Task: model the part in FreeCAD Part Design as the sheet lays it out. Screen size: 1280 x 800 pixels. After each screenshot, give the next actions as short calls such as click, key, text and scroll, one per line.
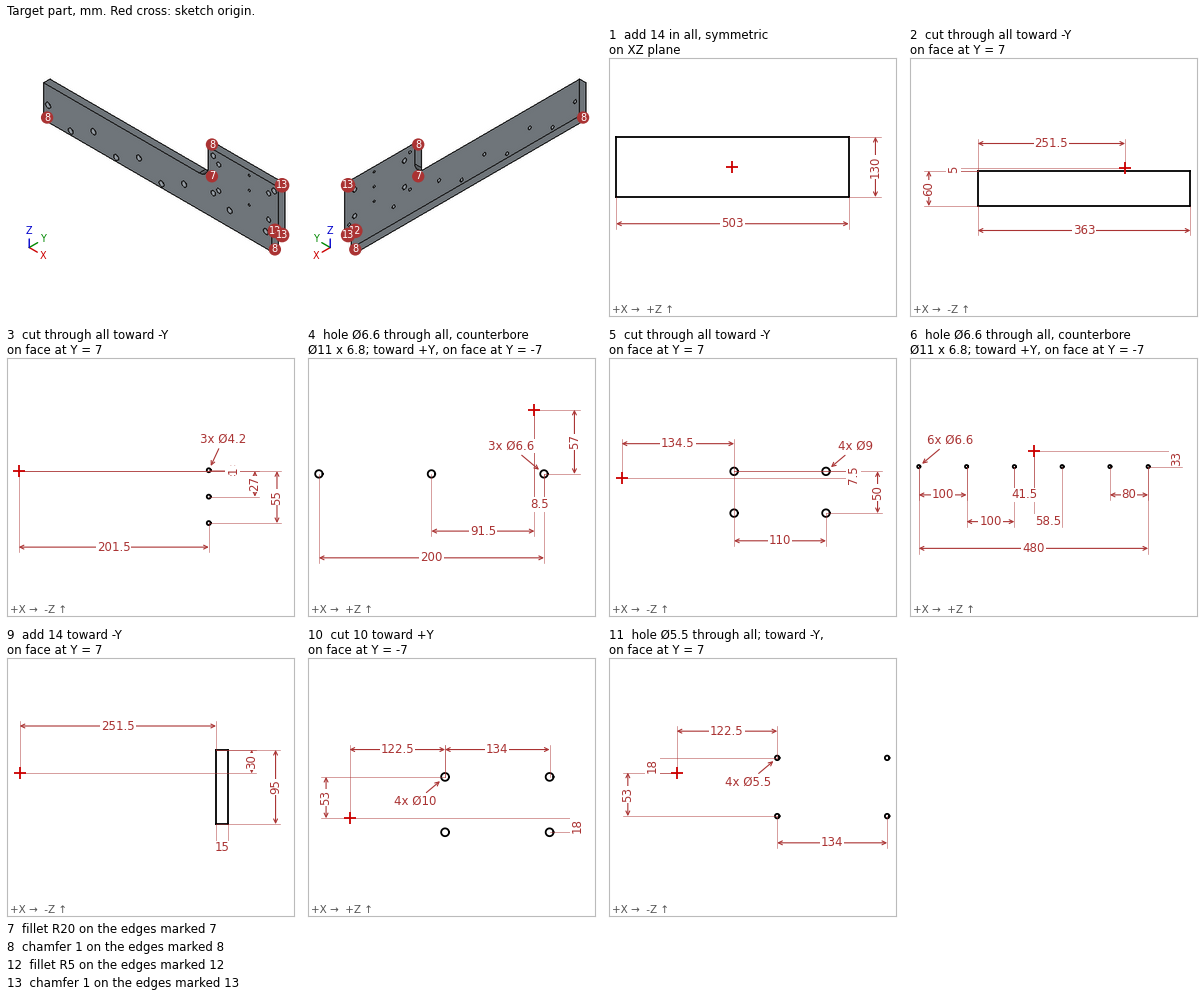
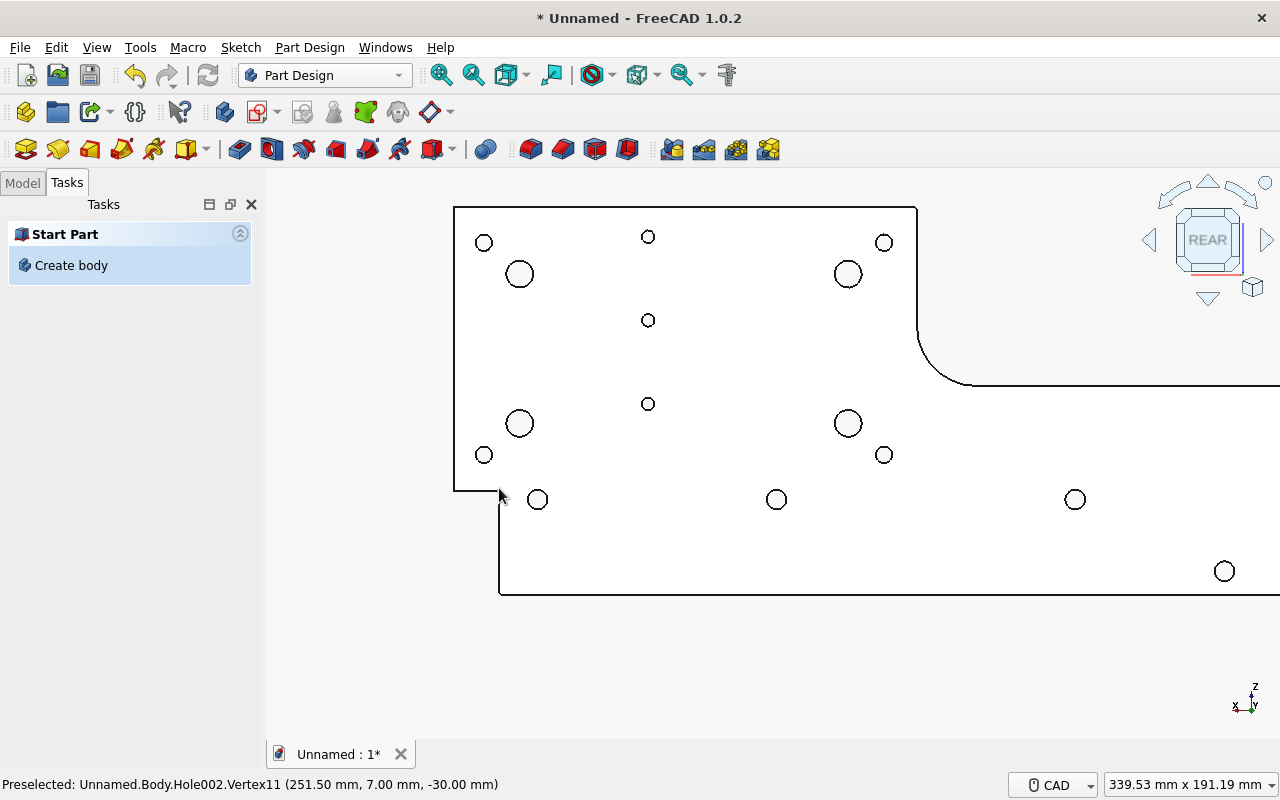
click(442, 76)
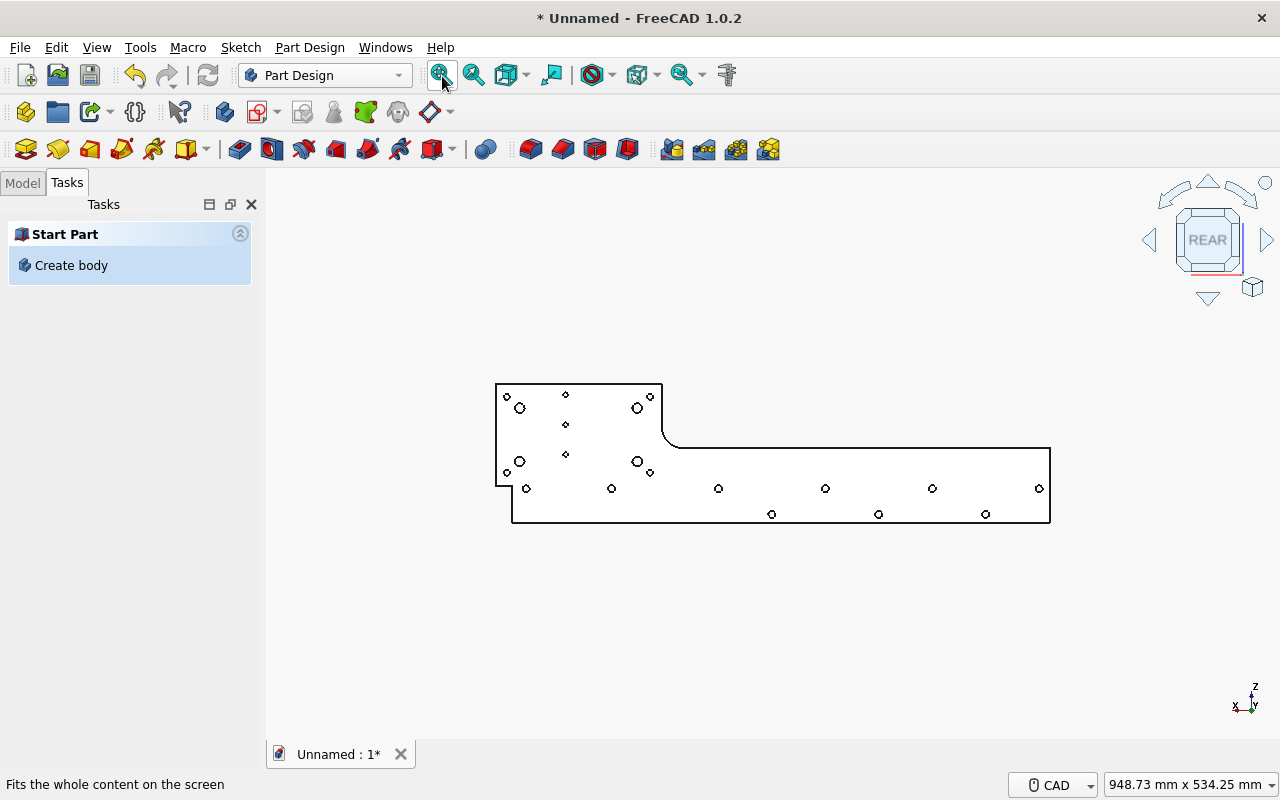
key(0)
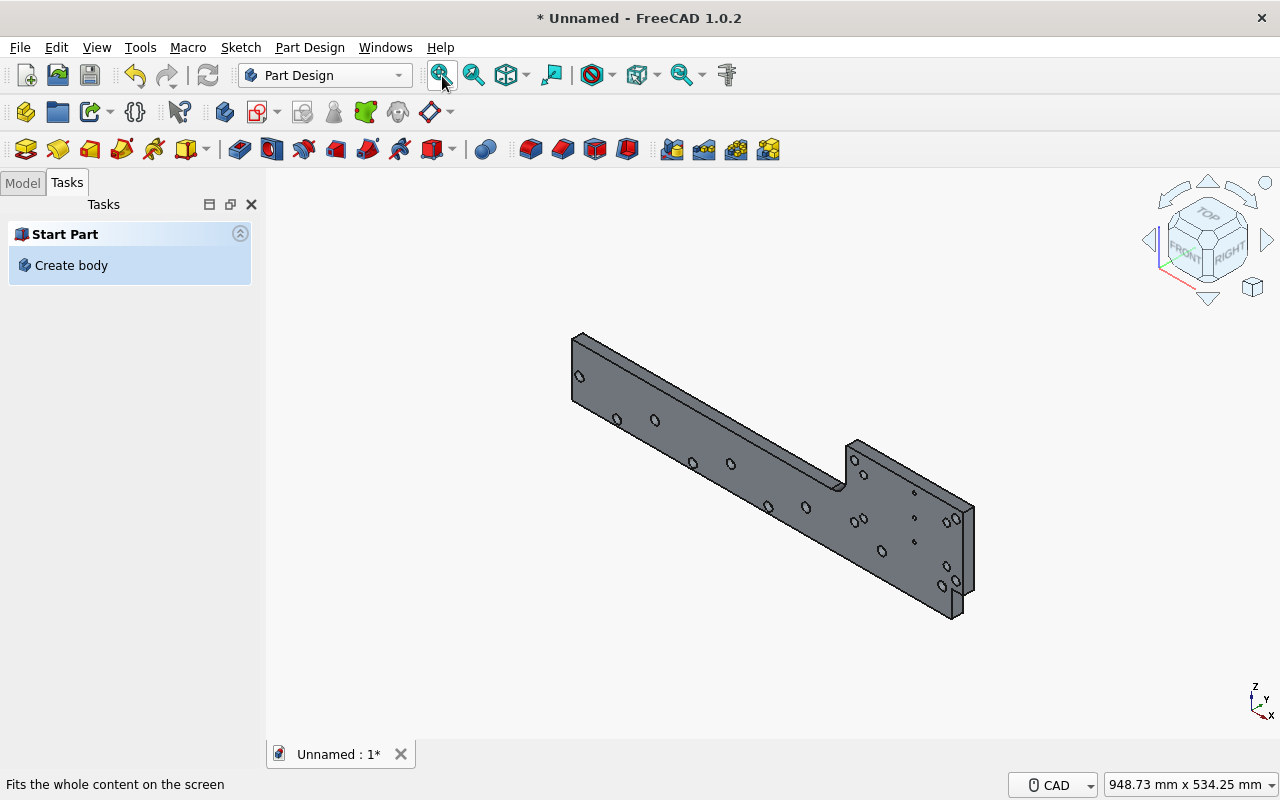
scroll(957, 585, up, 5)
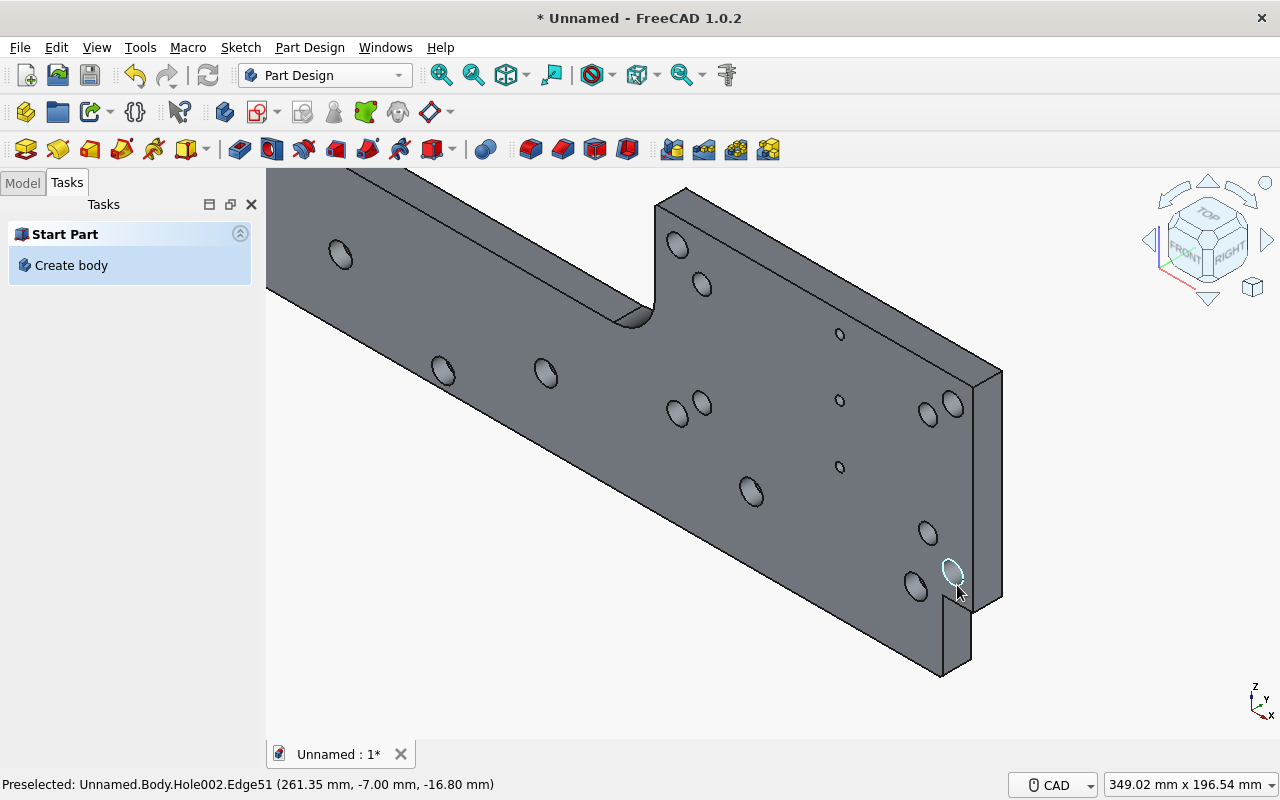
click(442, 76)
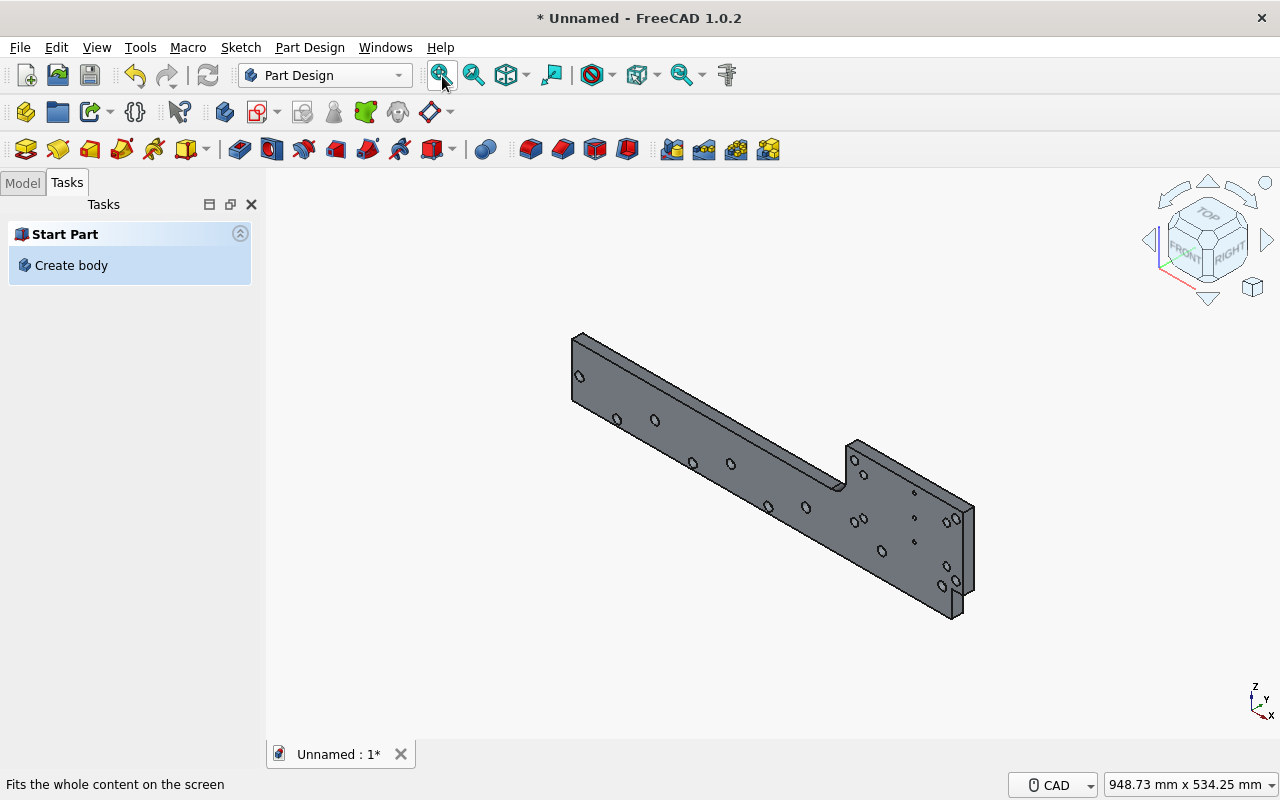
key(2)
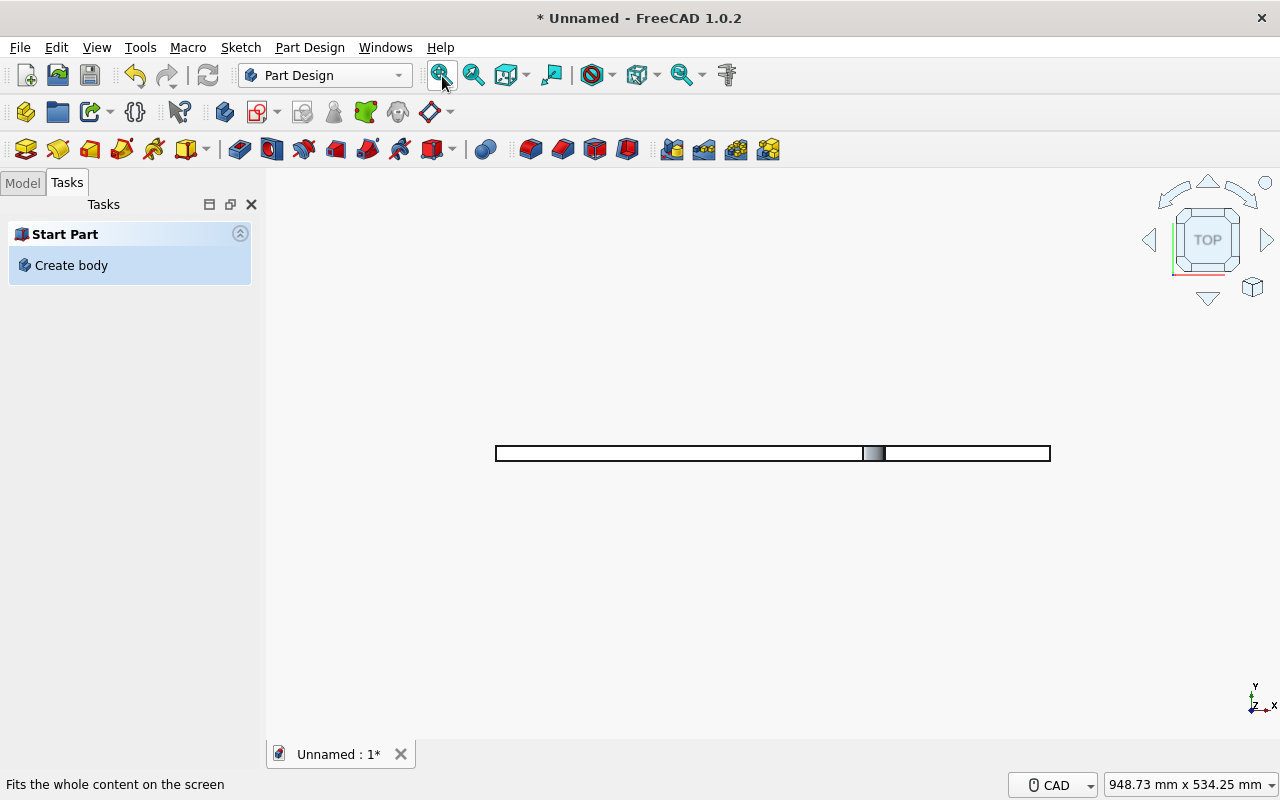
scroll(1034, 452, up, 5)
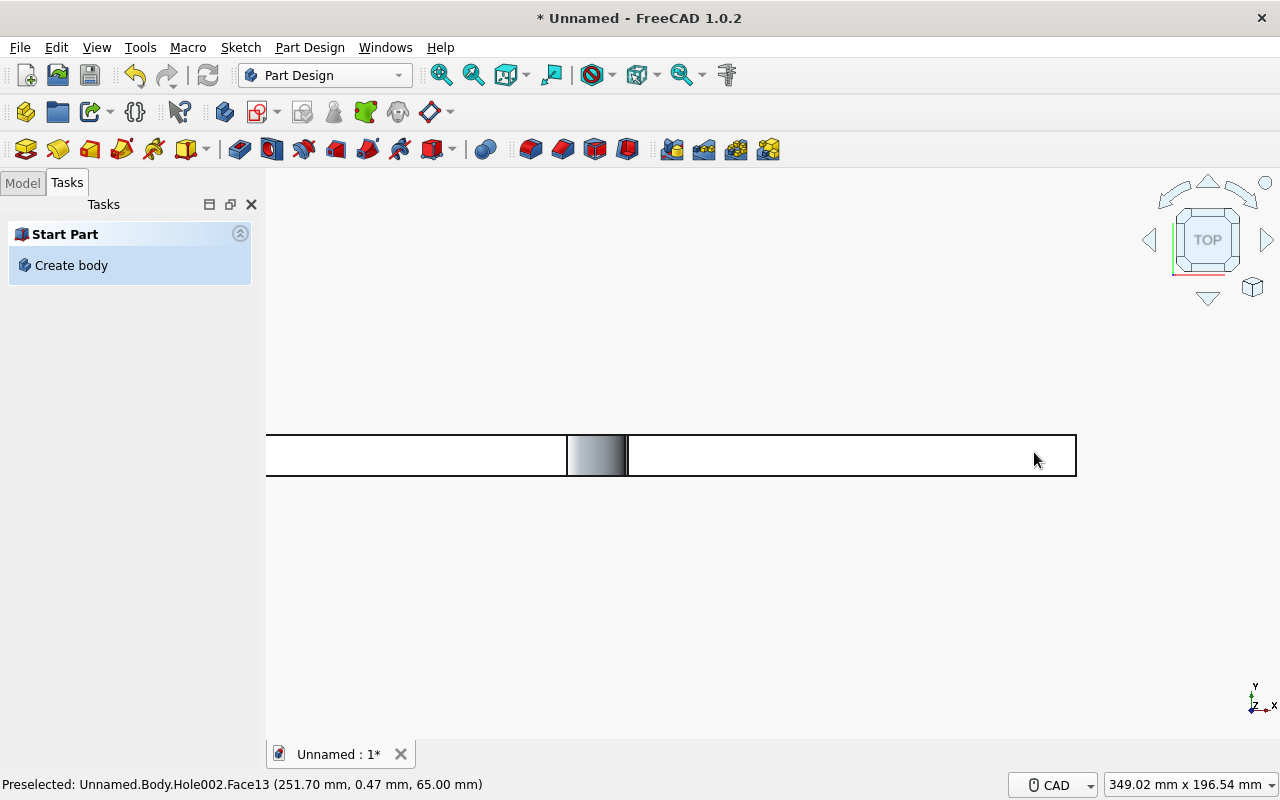
key(v)
key(f)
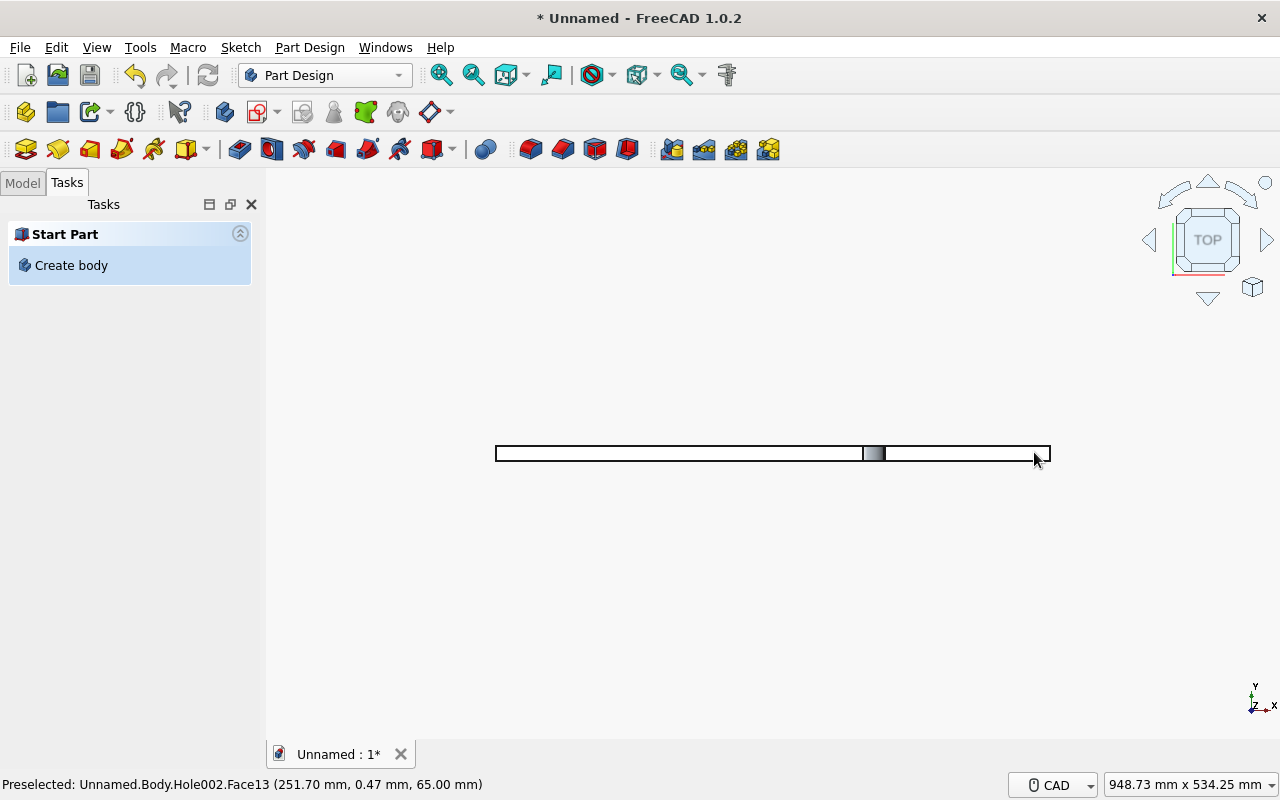
key(1)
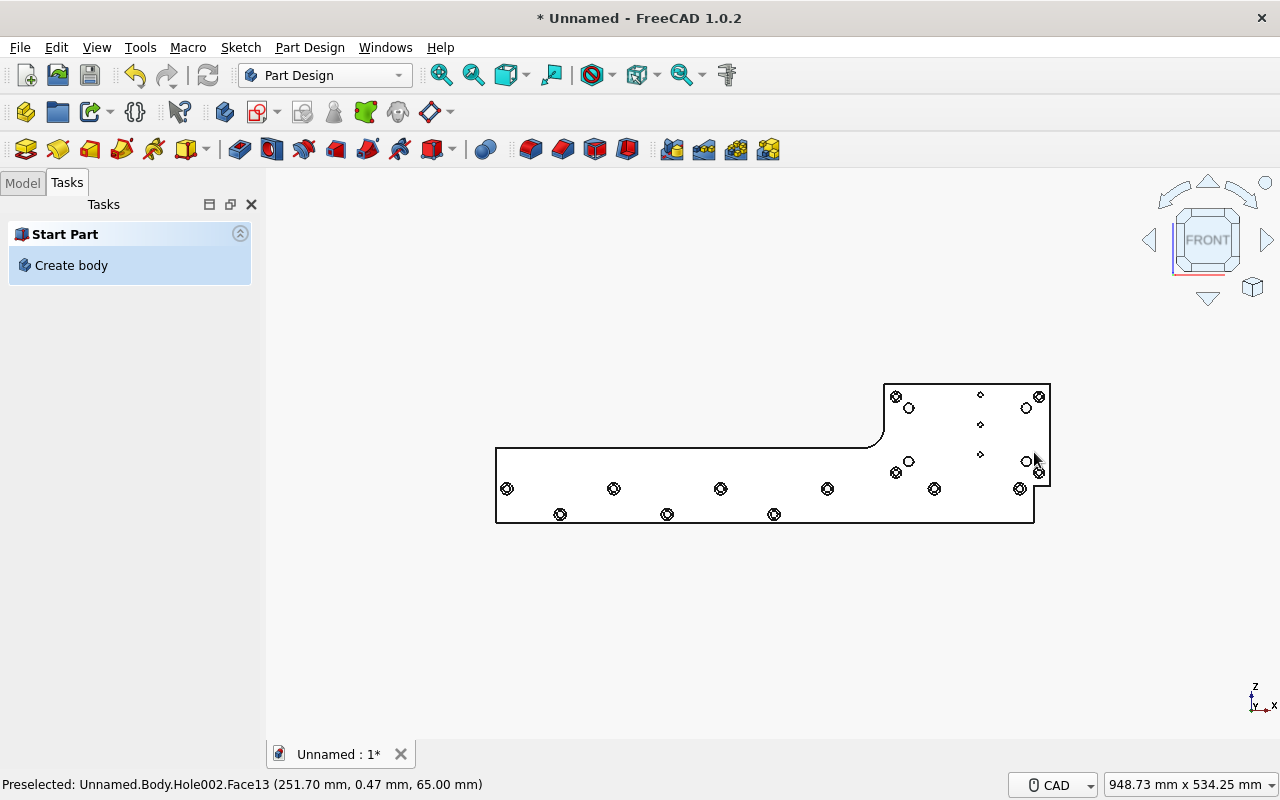
scroll(1034, 485, up, 5)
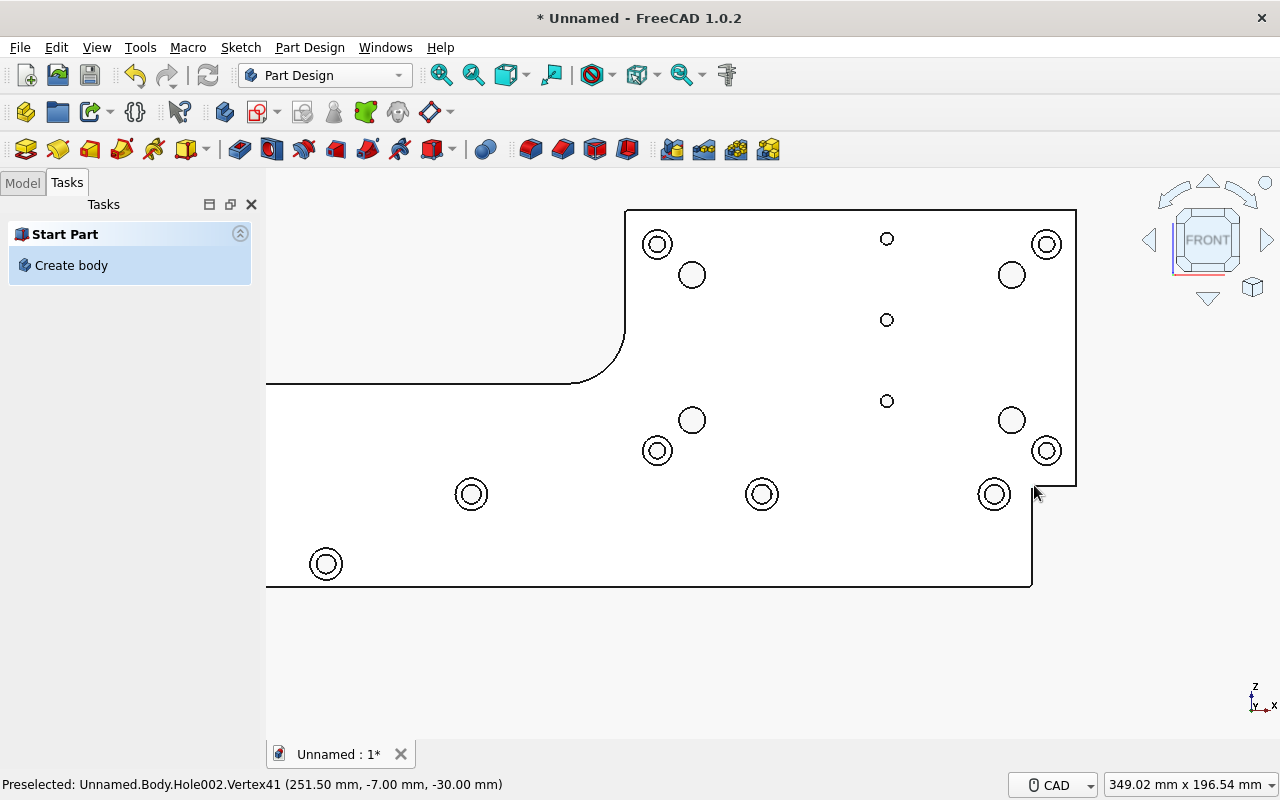
key(v)
key(f)